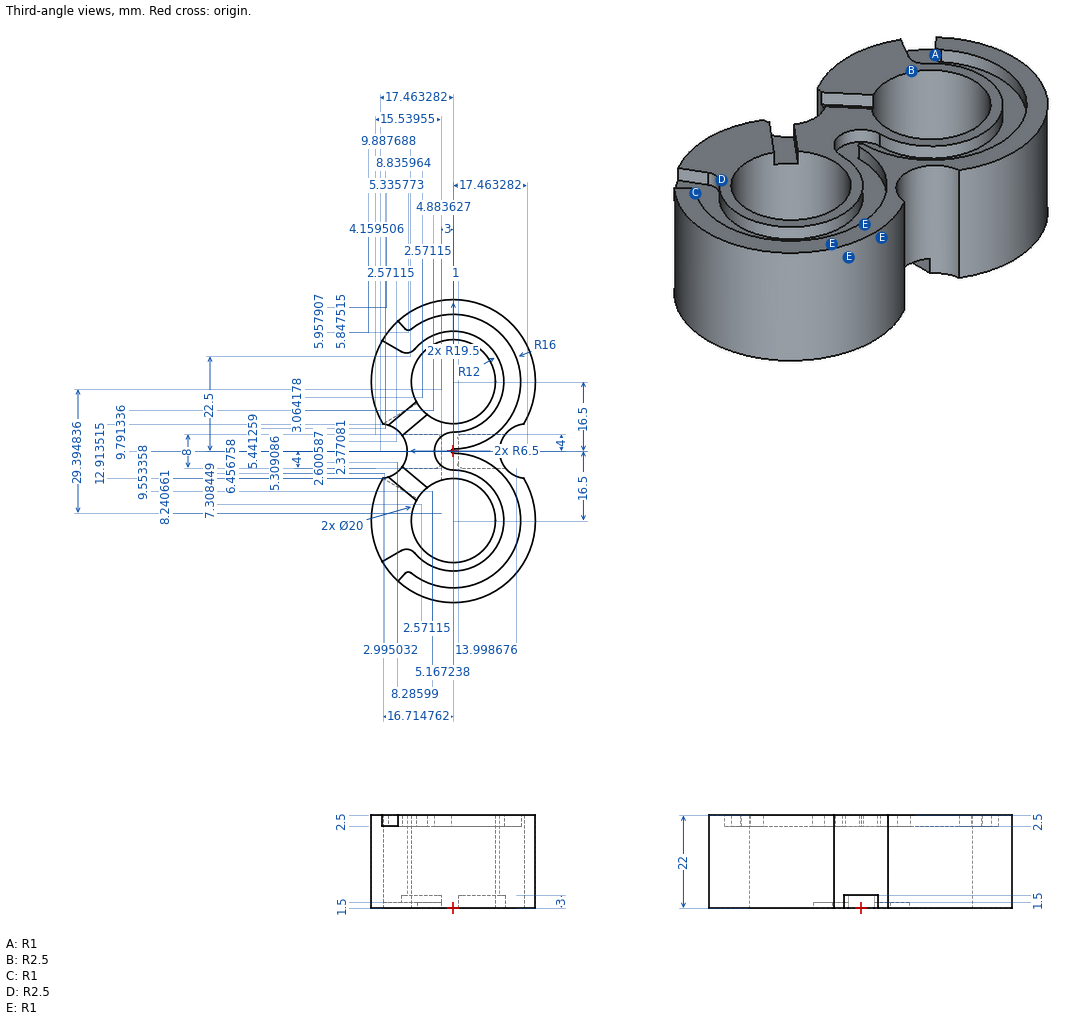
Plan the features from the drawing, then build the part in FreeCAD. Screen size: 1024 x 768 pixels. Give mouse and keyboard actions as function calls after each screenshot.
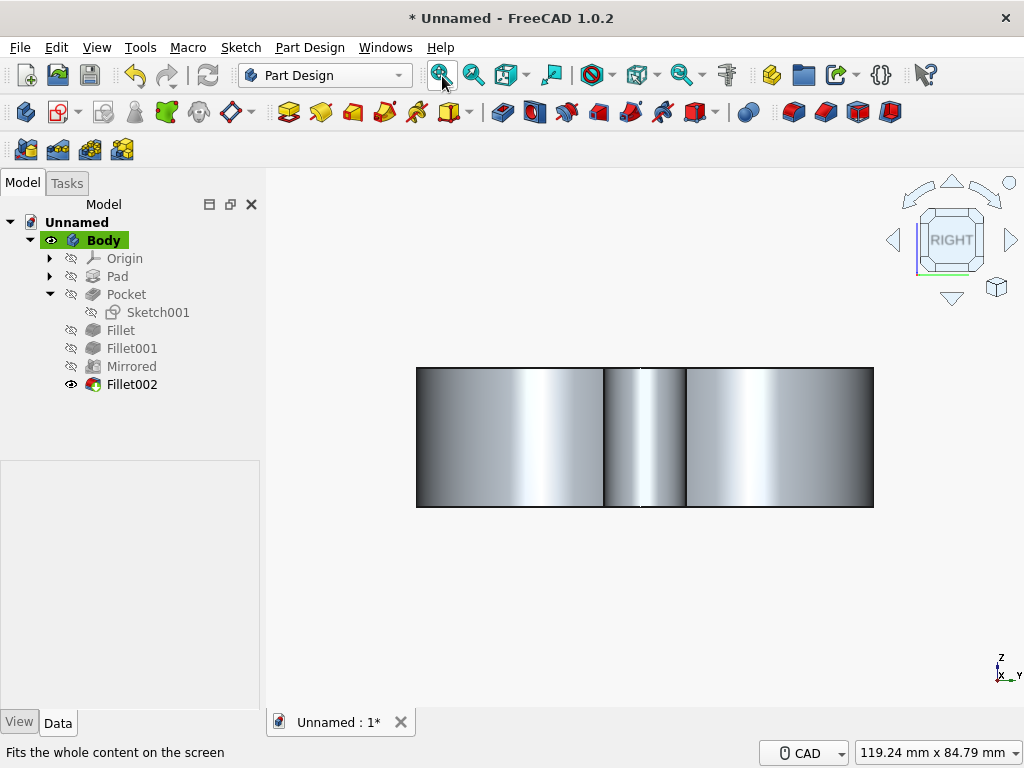
key(5)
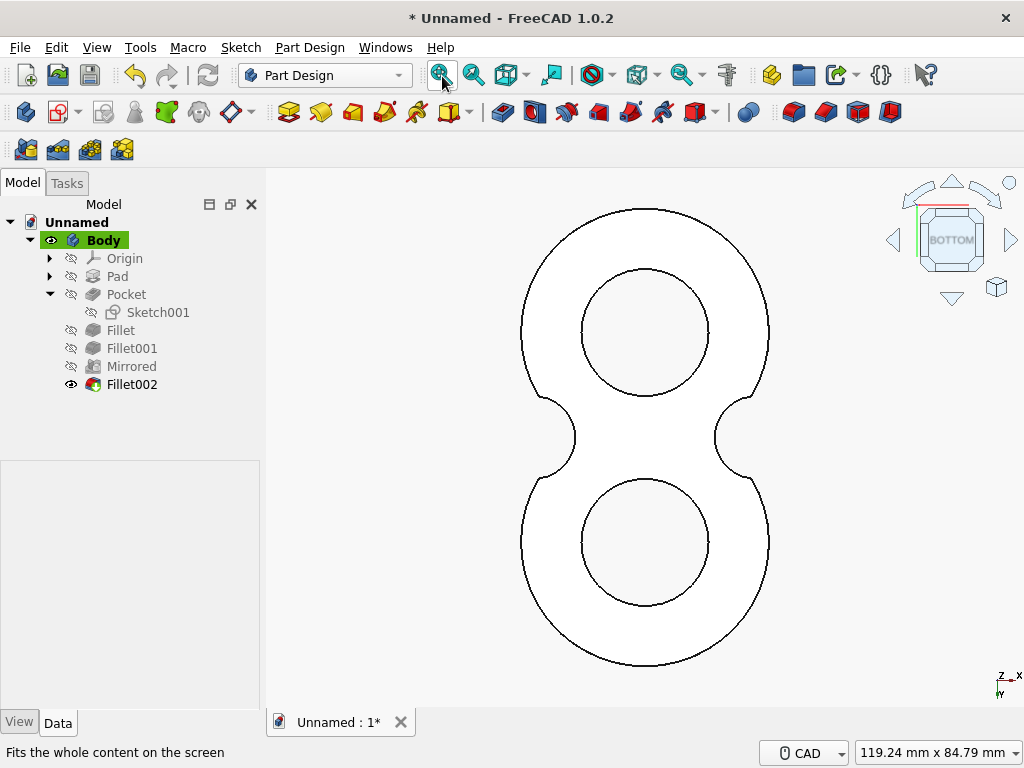
scroll(579, 293, up, 5)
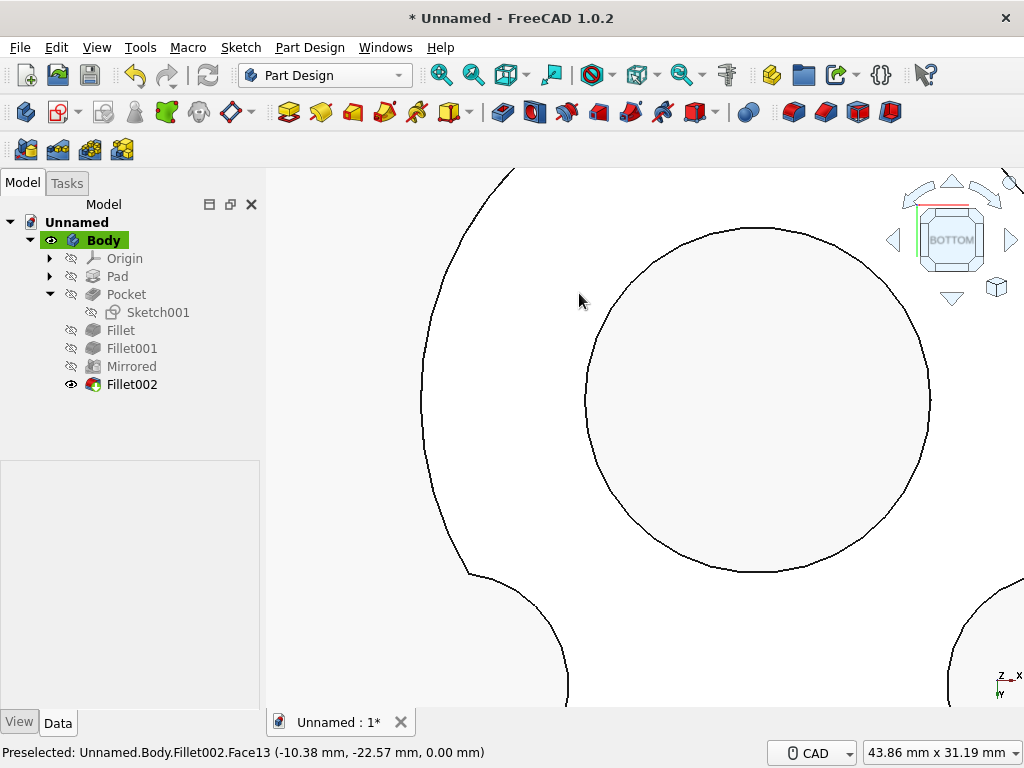
key(v)
key(f)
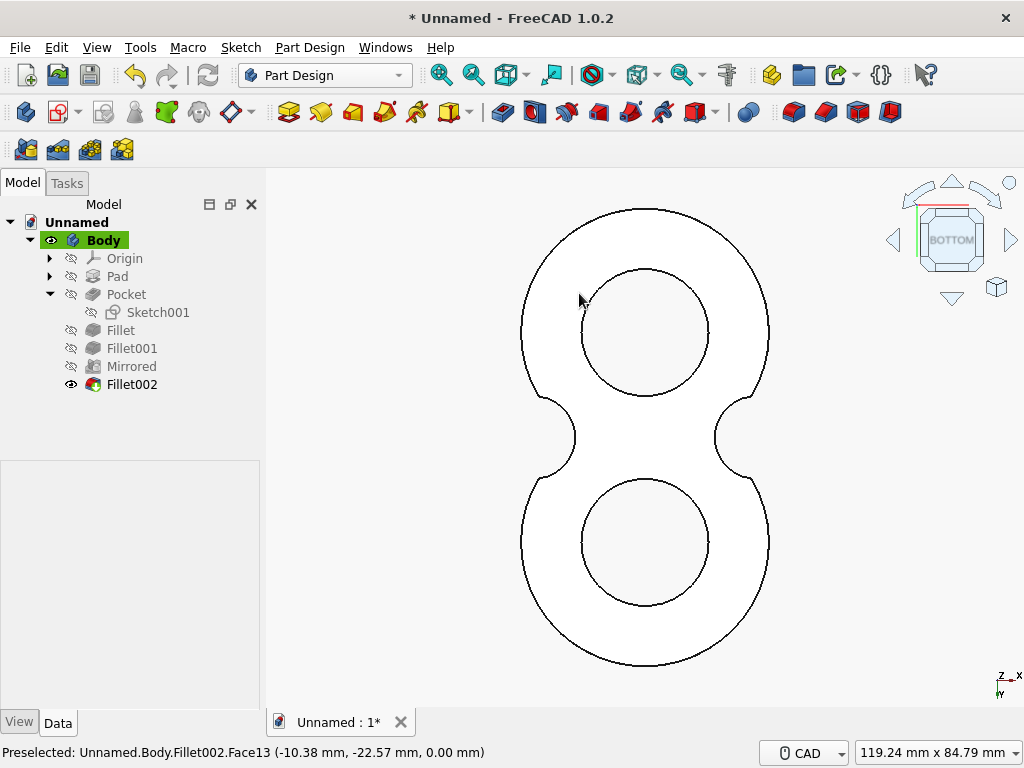
key(4)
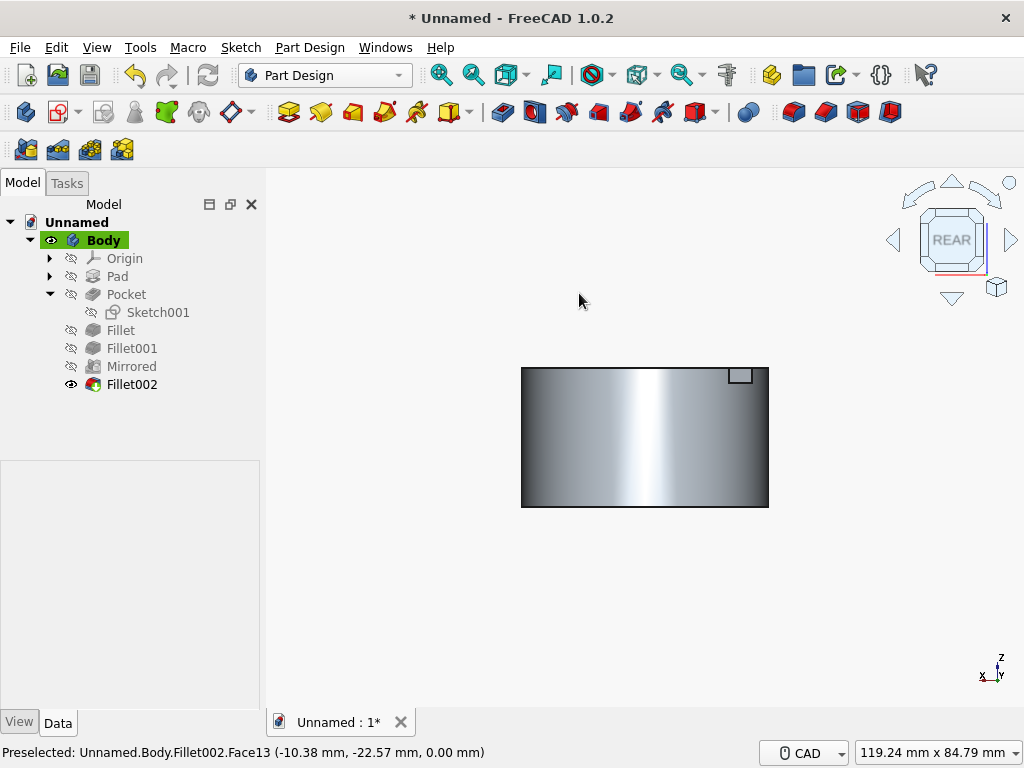
key(v)
key(f)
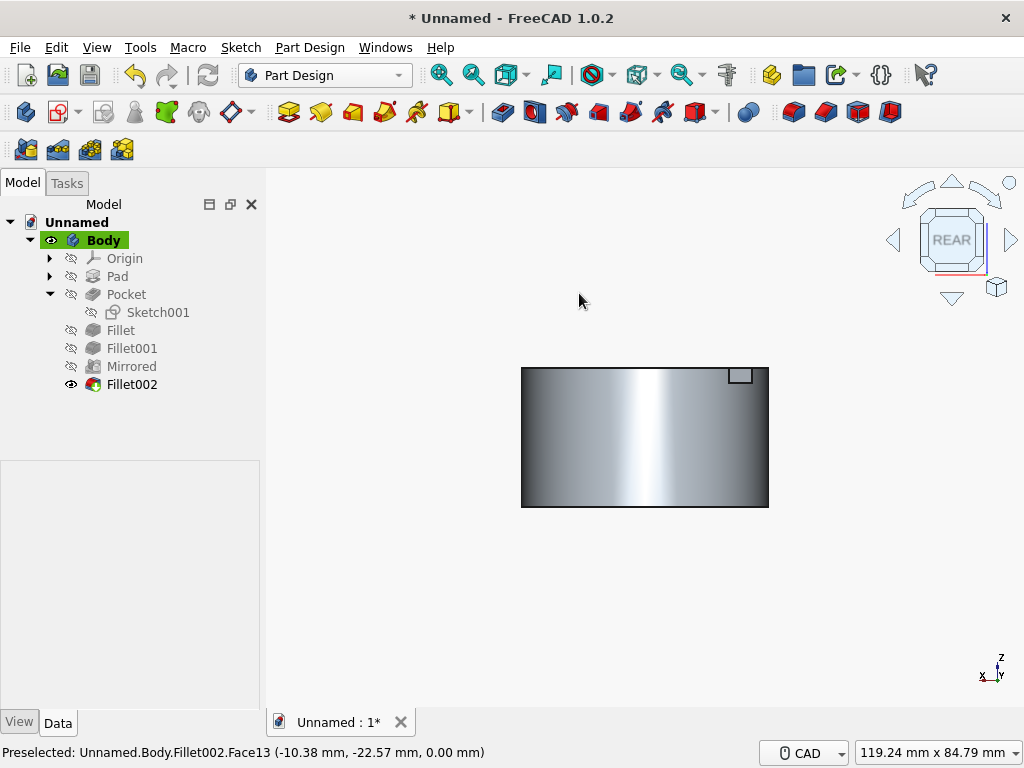
scroll(711, 375, up, 5)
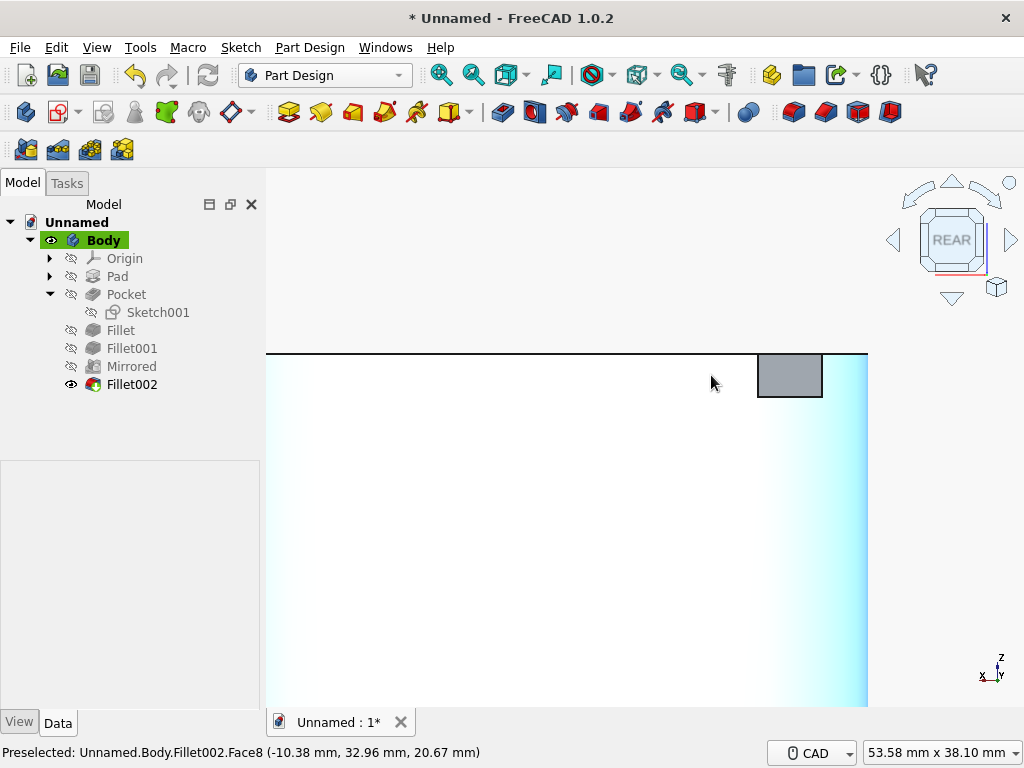
key(v)
key(f)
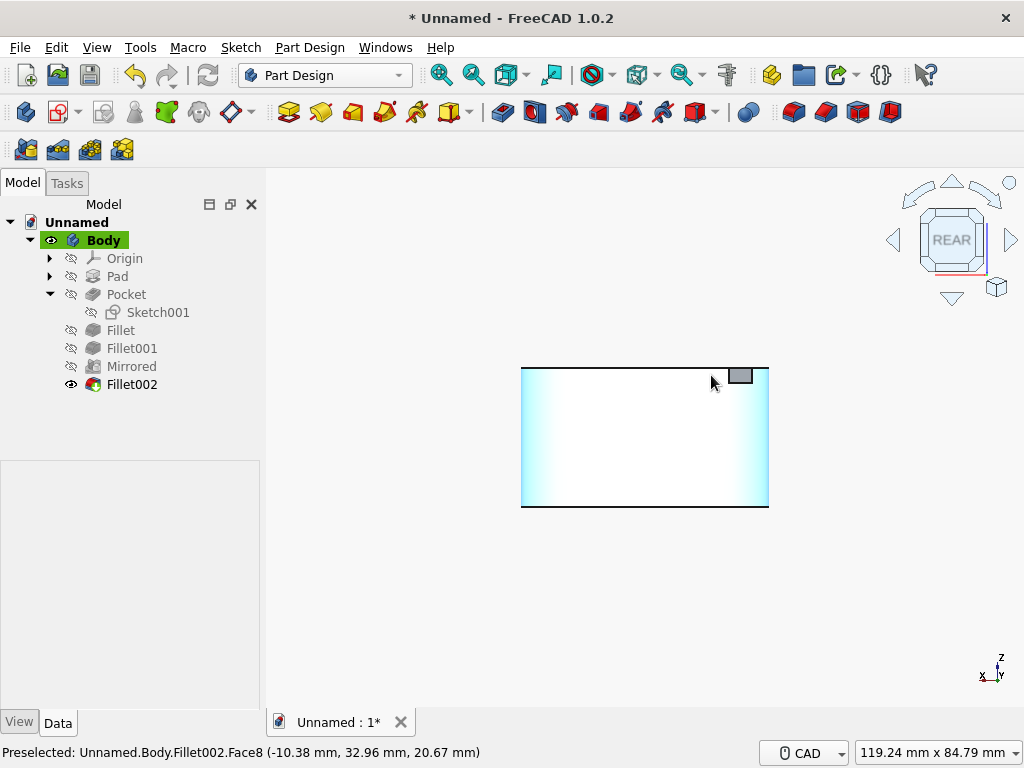
key(6)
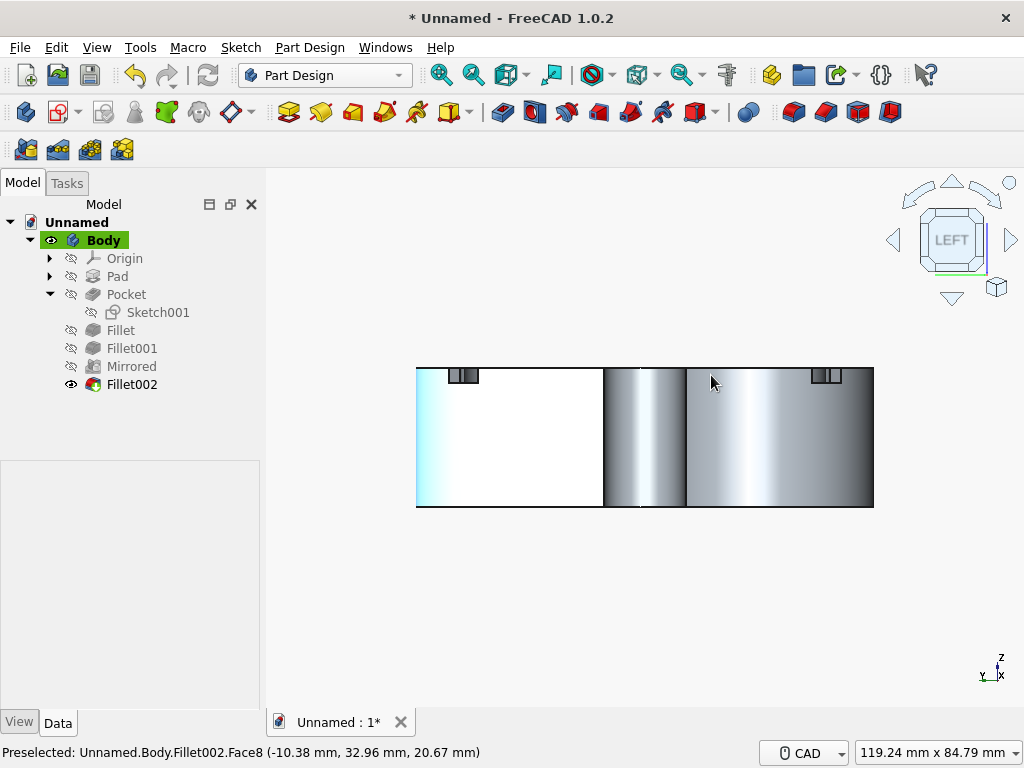
scroll(788, 375, up, 5)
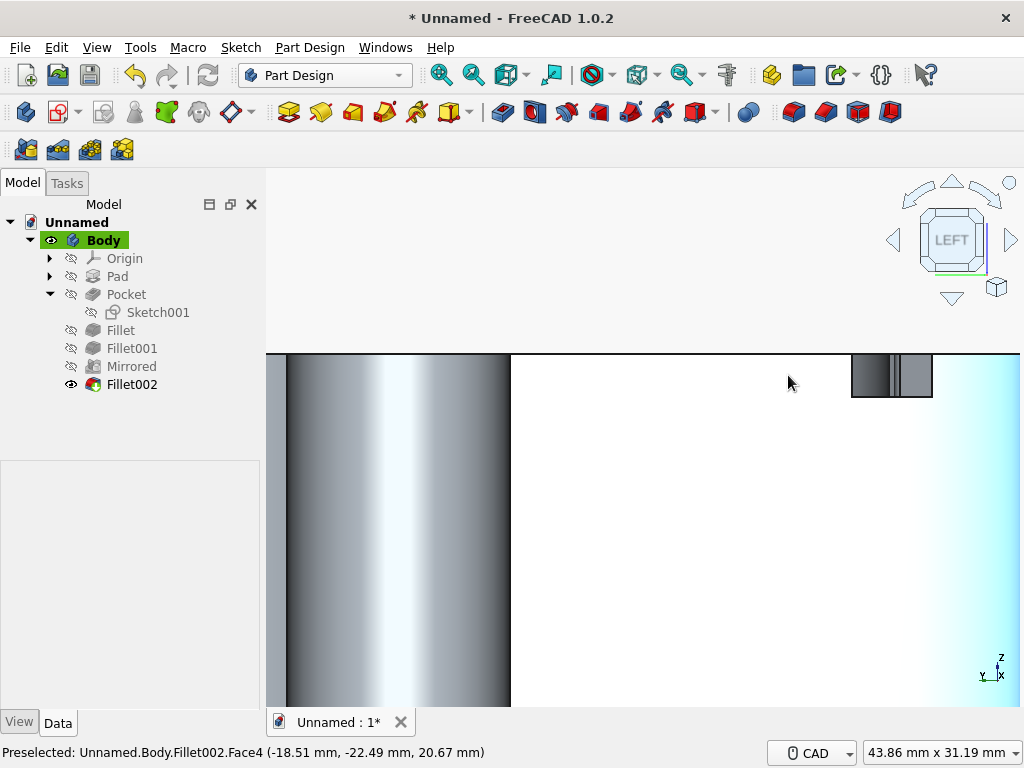
key(v)
key(f)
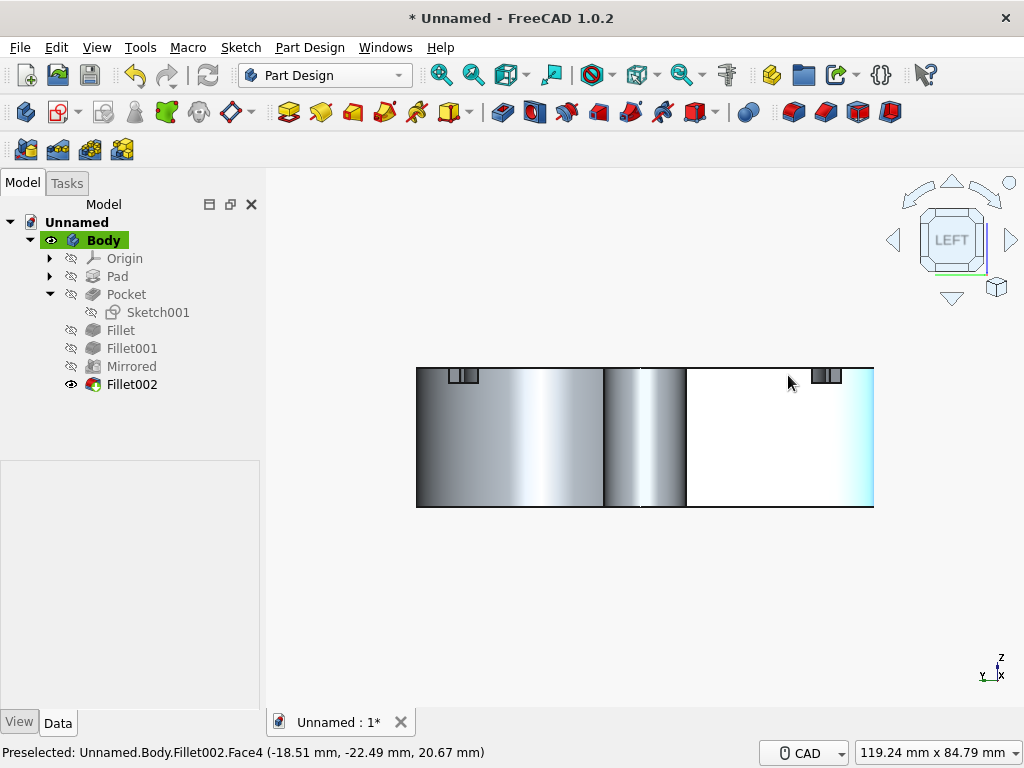
key(v)
key(3)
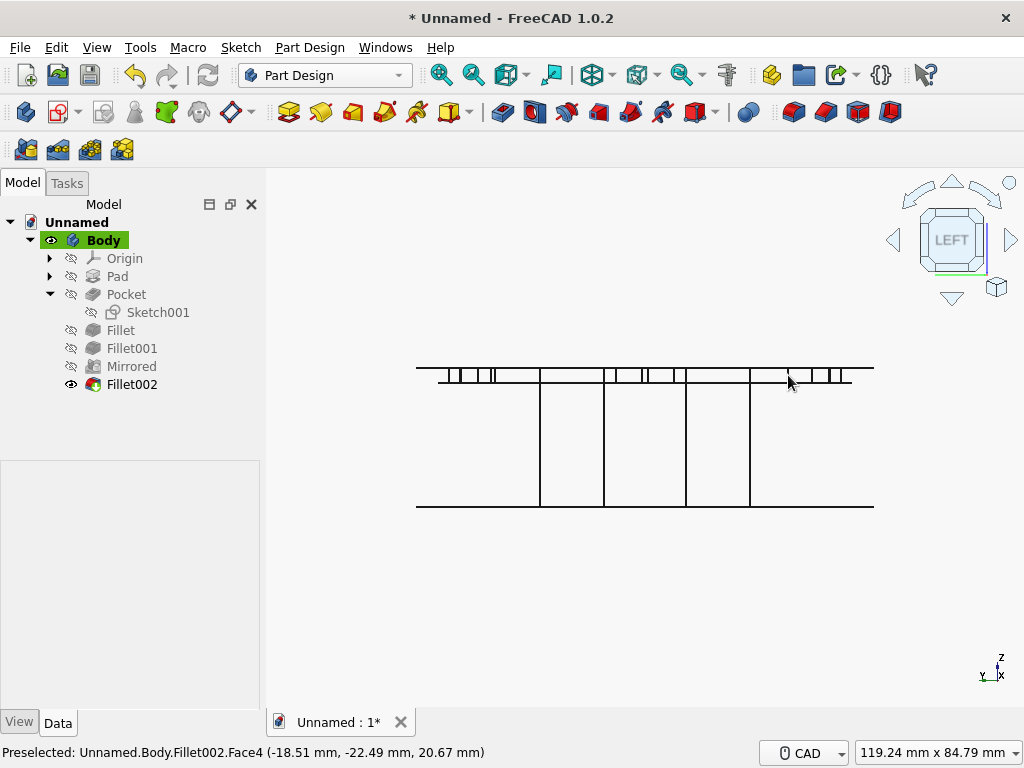
key(0)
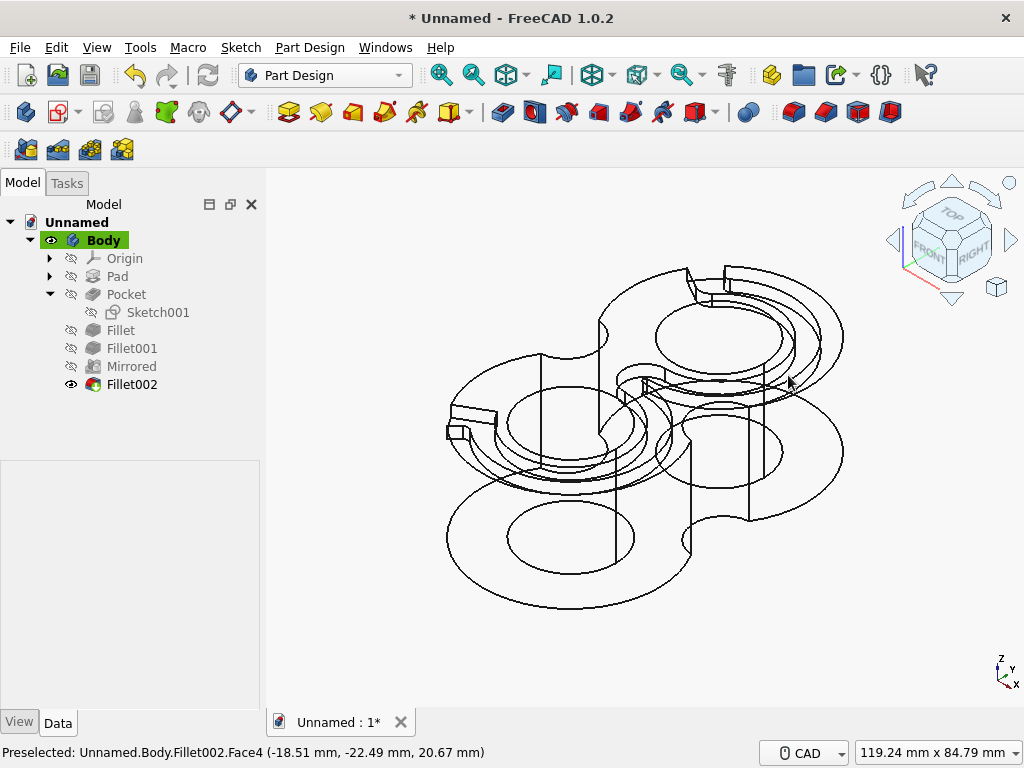
scroll(497, 417, up, 6)